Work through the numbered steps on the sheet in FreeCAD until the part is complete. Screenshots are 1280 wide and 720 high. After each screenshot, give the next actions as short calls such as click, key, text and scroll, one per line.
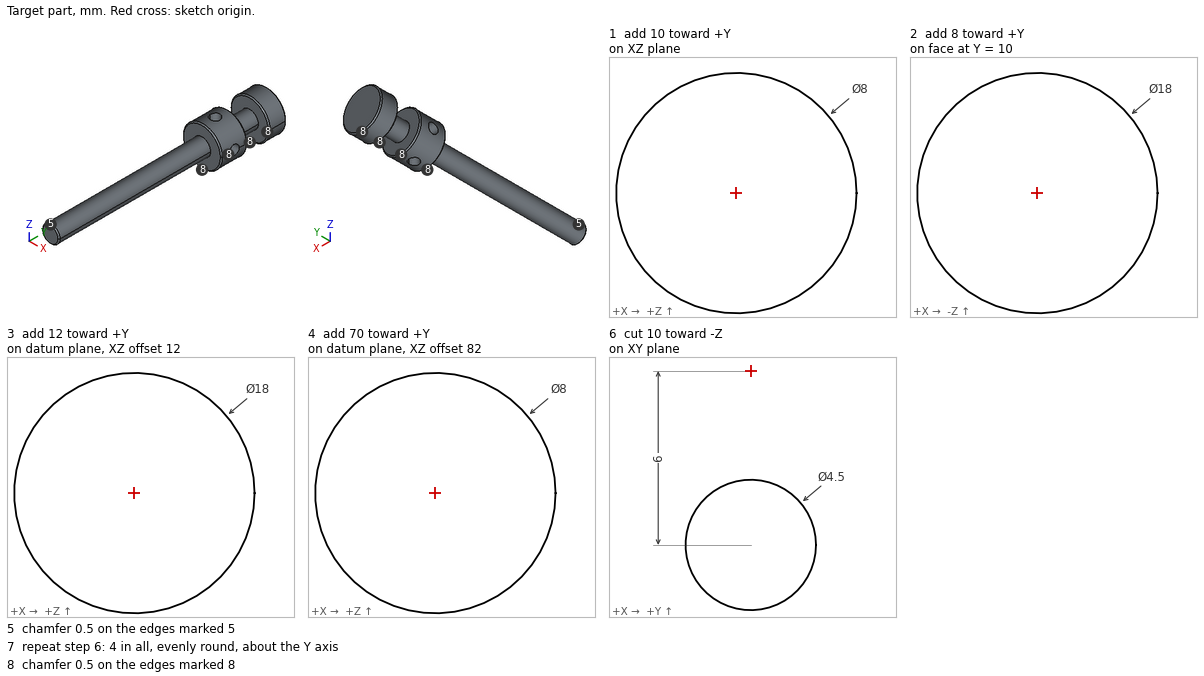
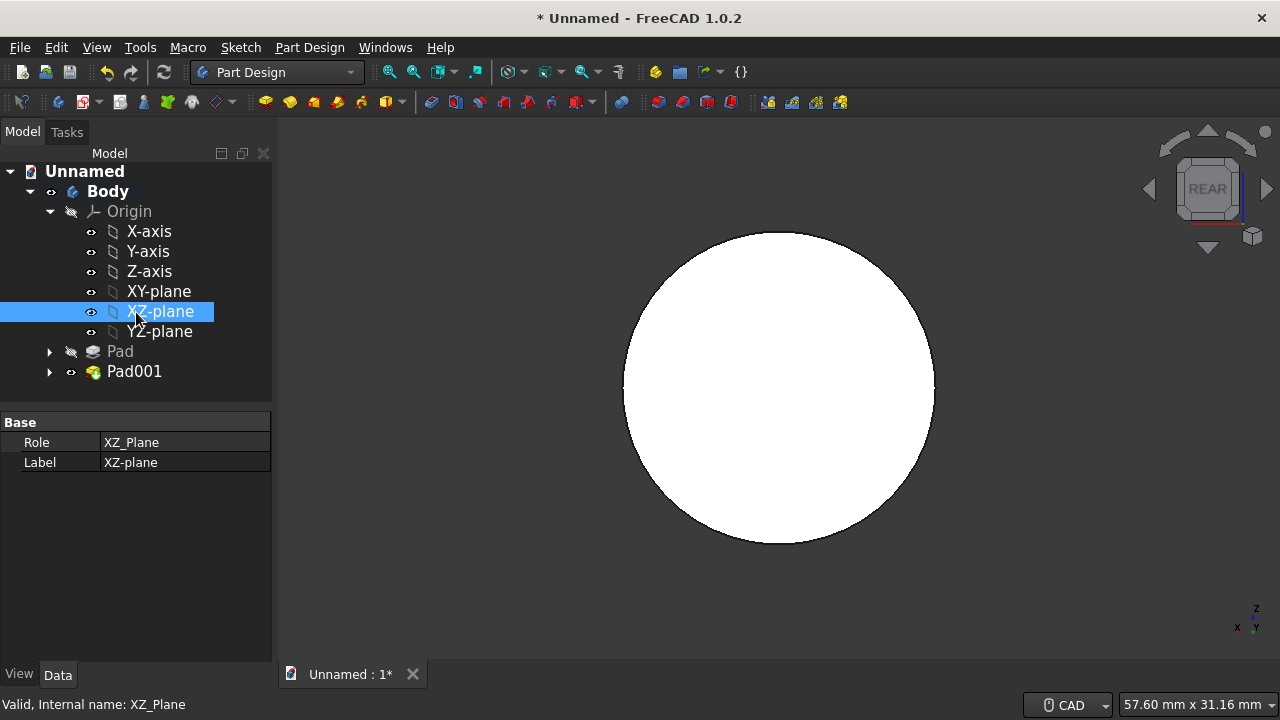
click(216, 102)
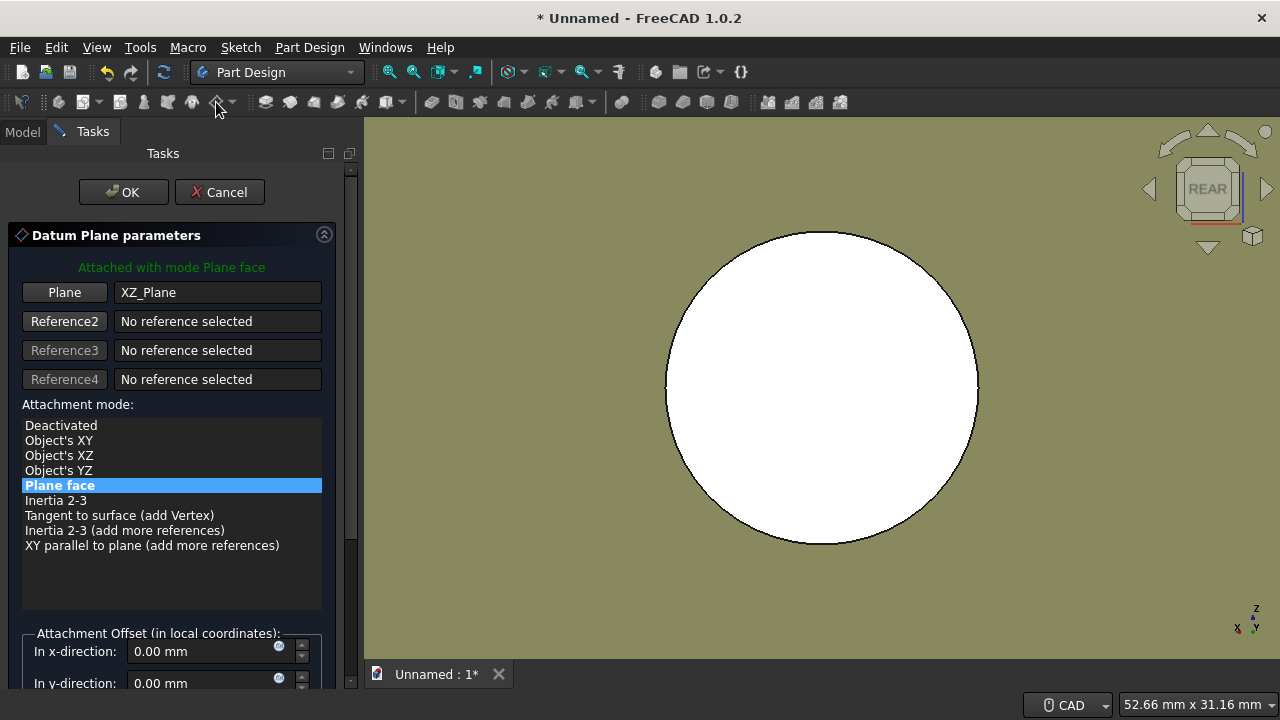
scroll(351, 426, down, 2)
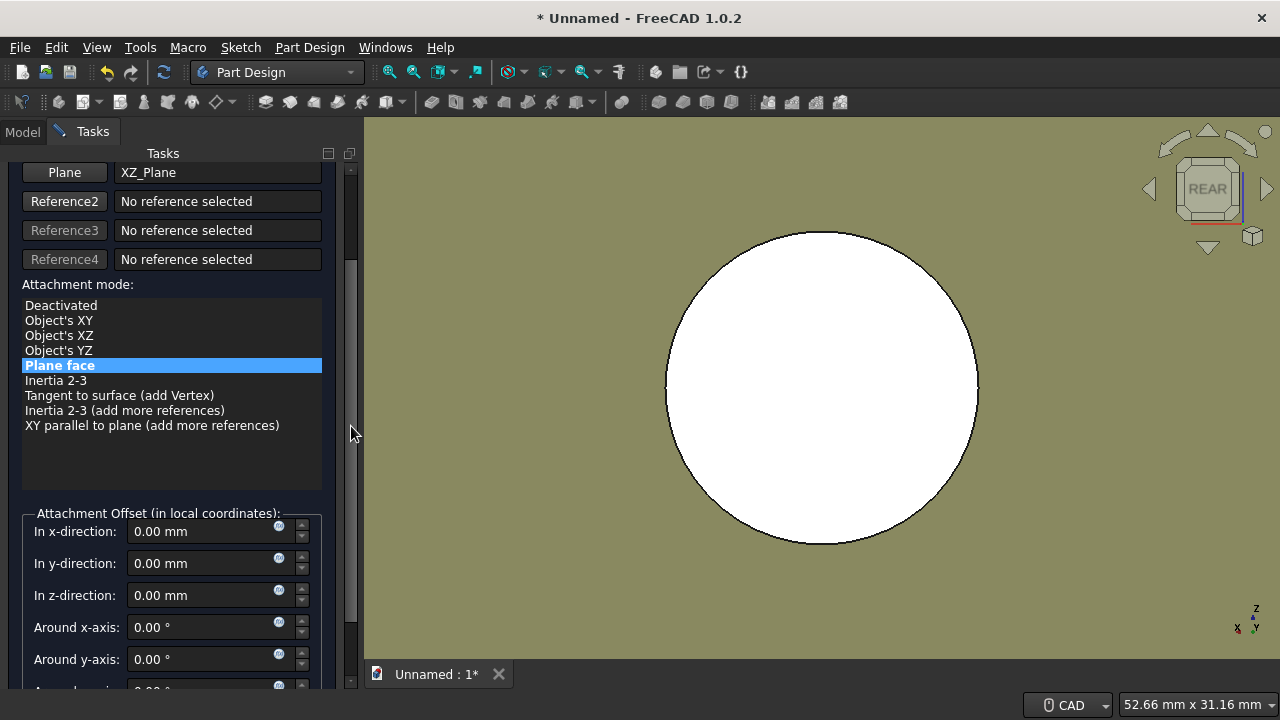
triple_click(210, 595)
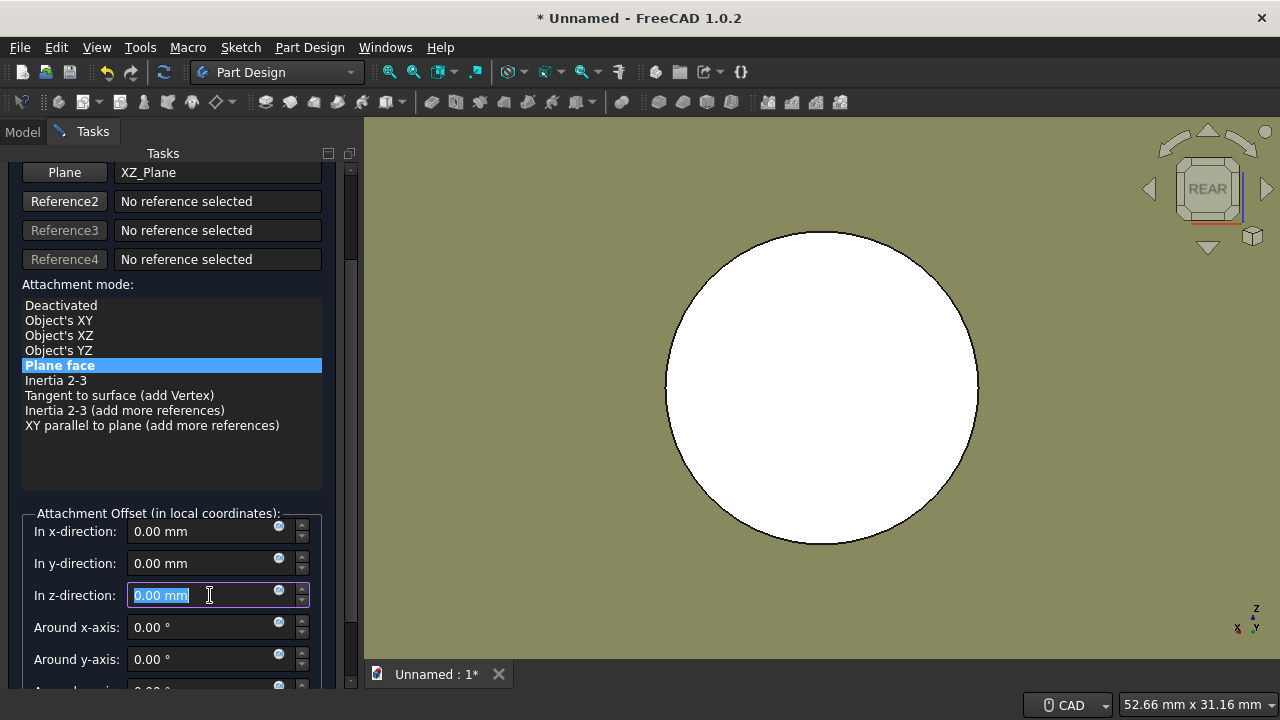
text(12)
key(Tab)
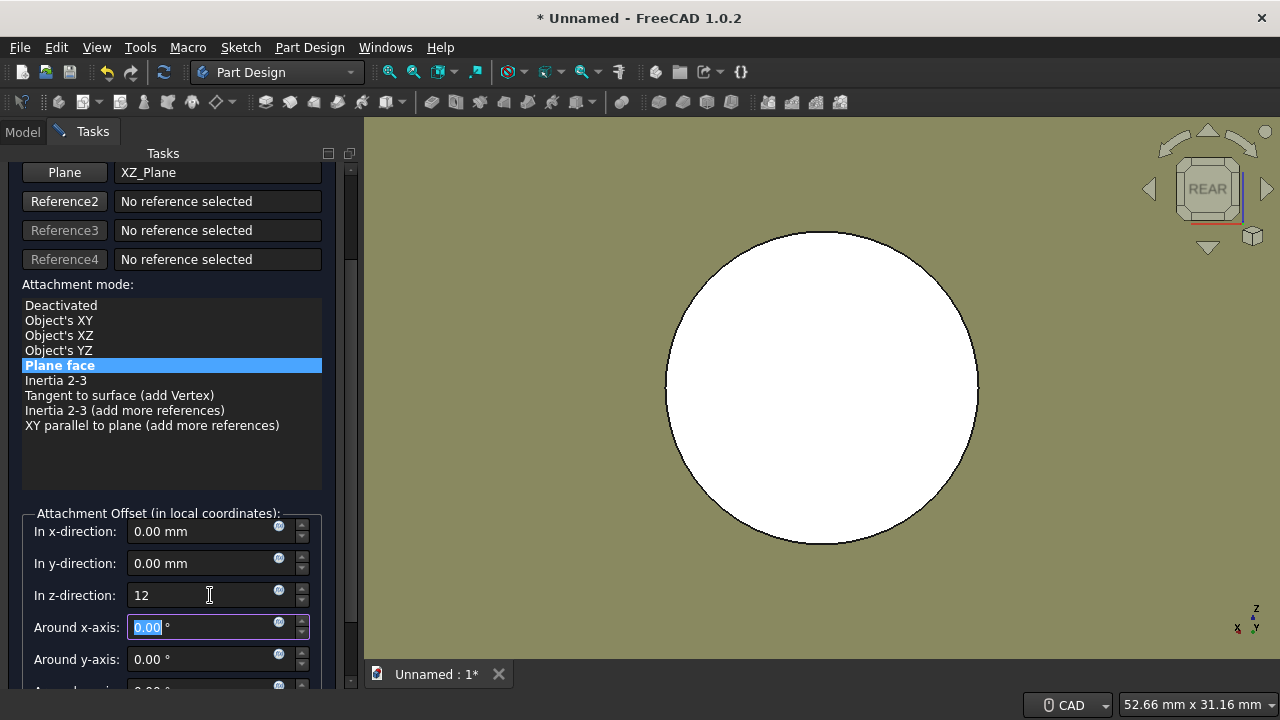
scroll(351, 426, up, 3)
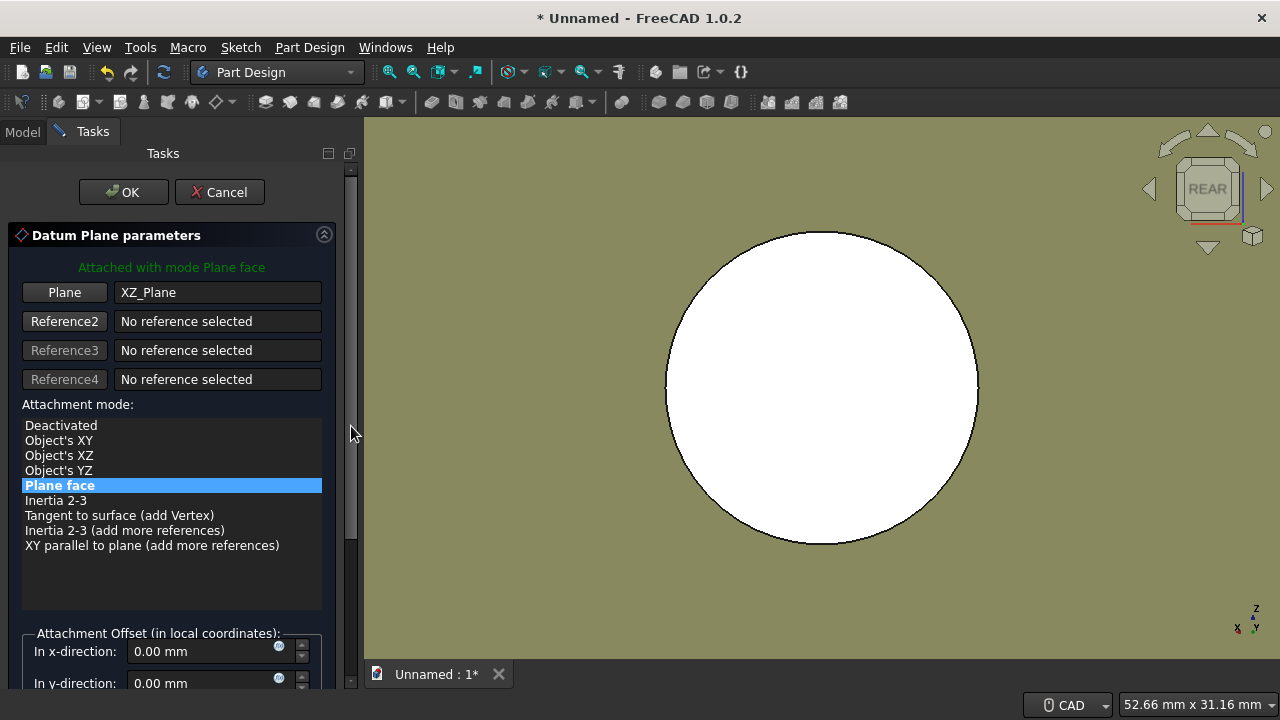
click(124, 192)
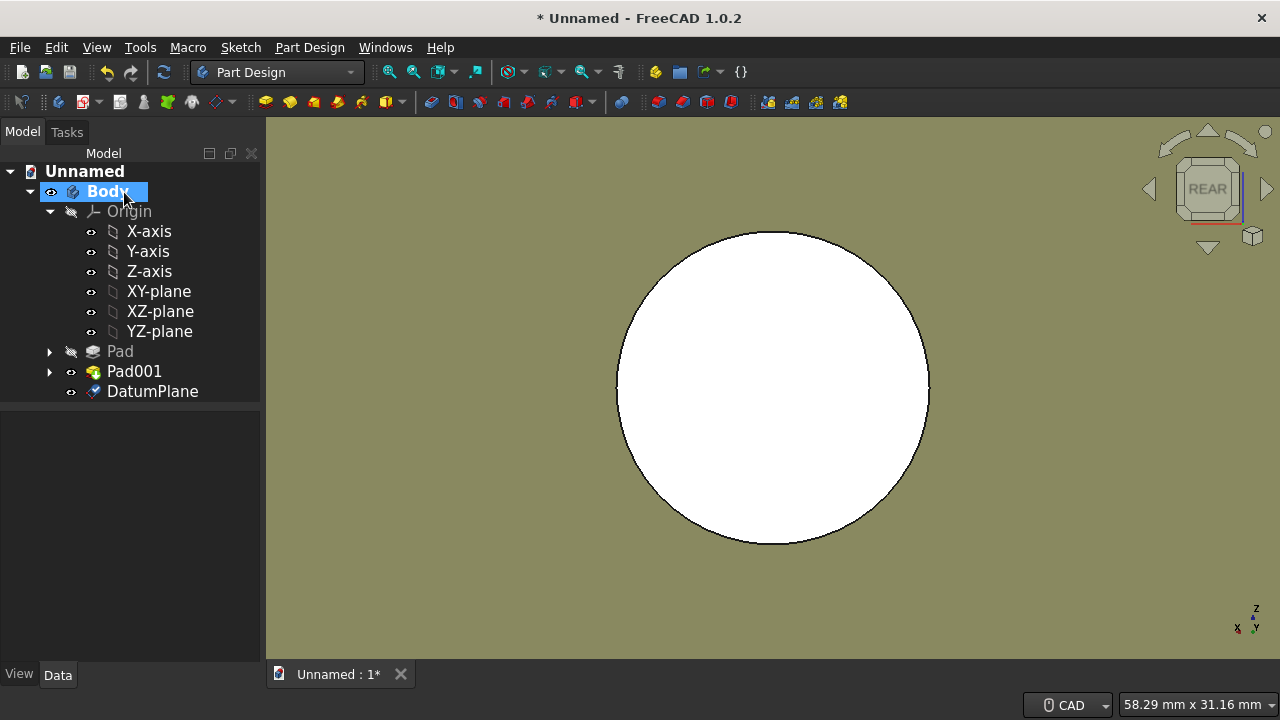
click(116, 392)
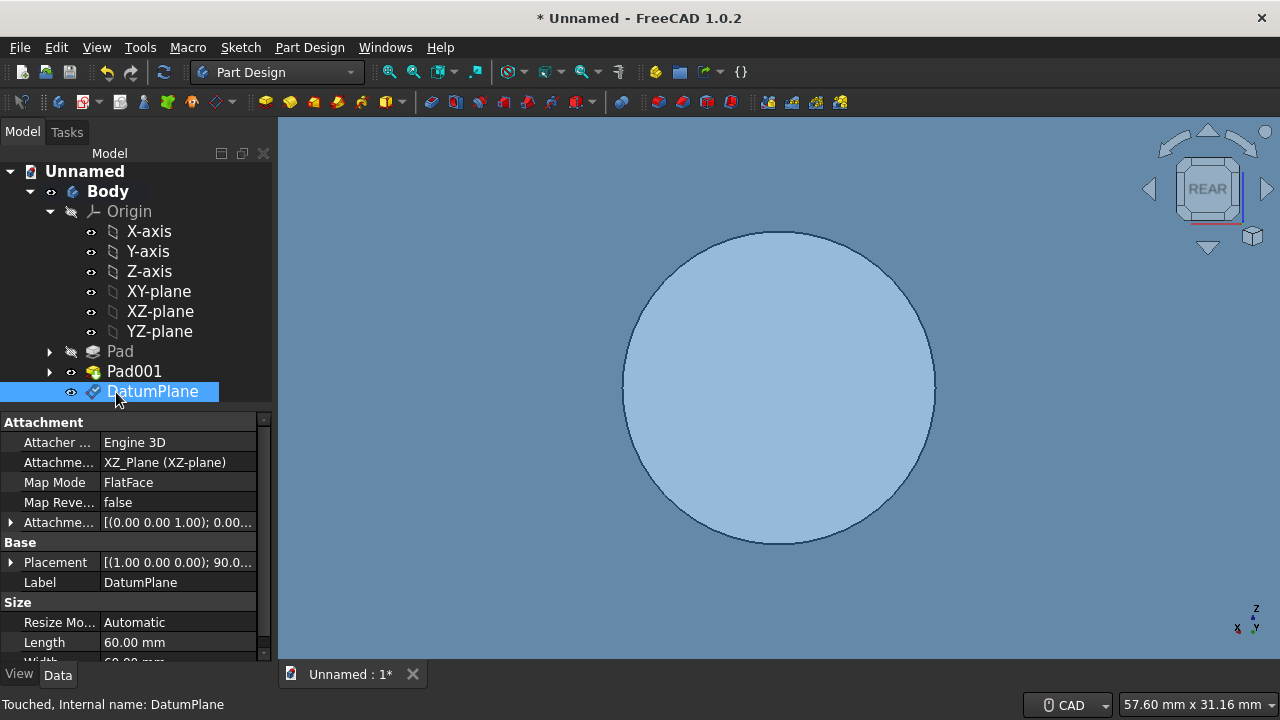
click(84, 102)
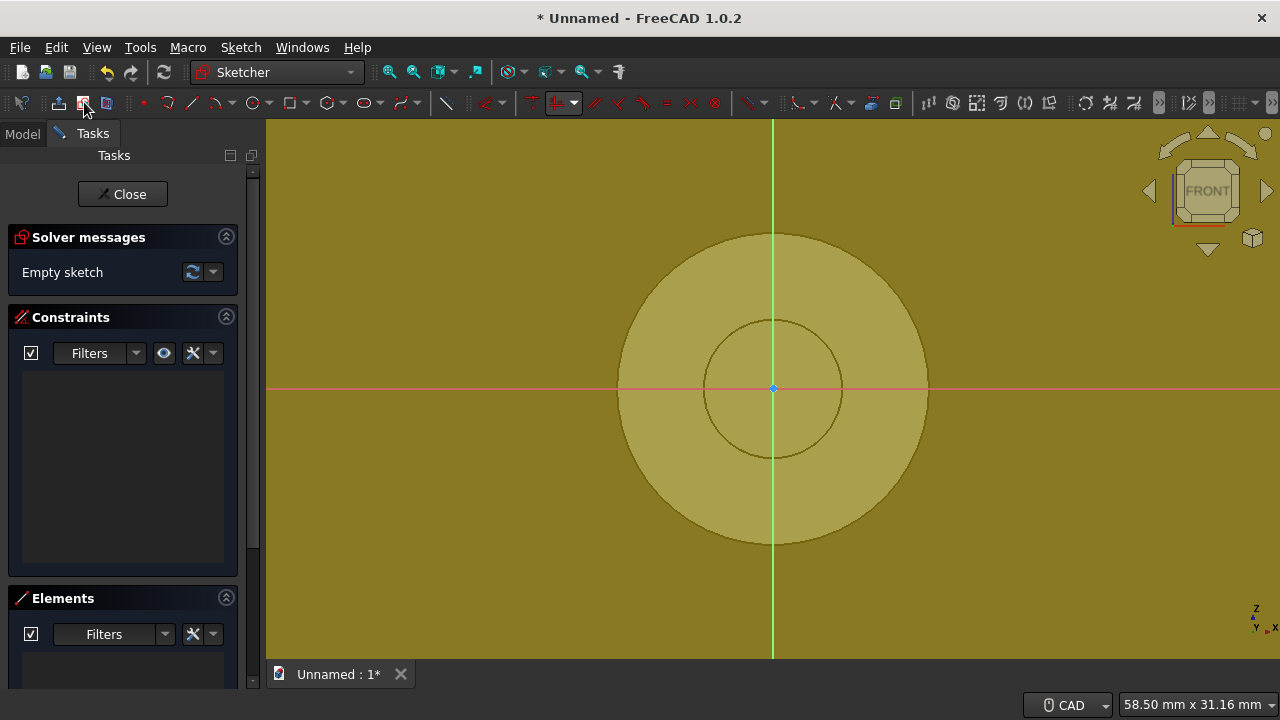
click(254, 104)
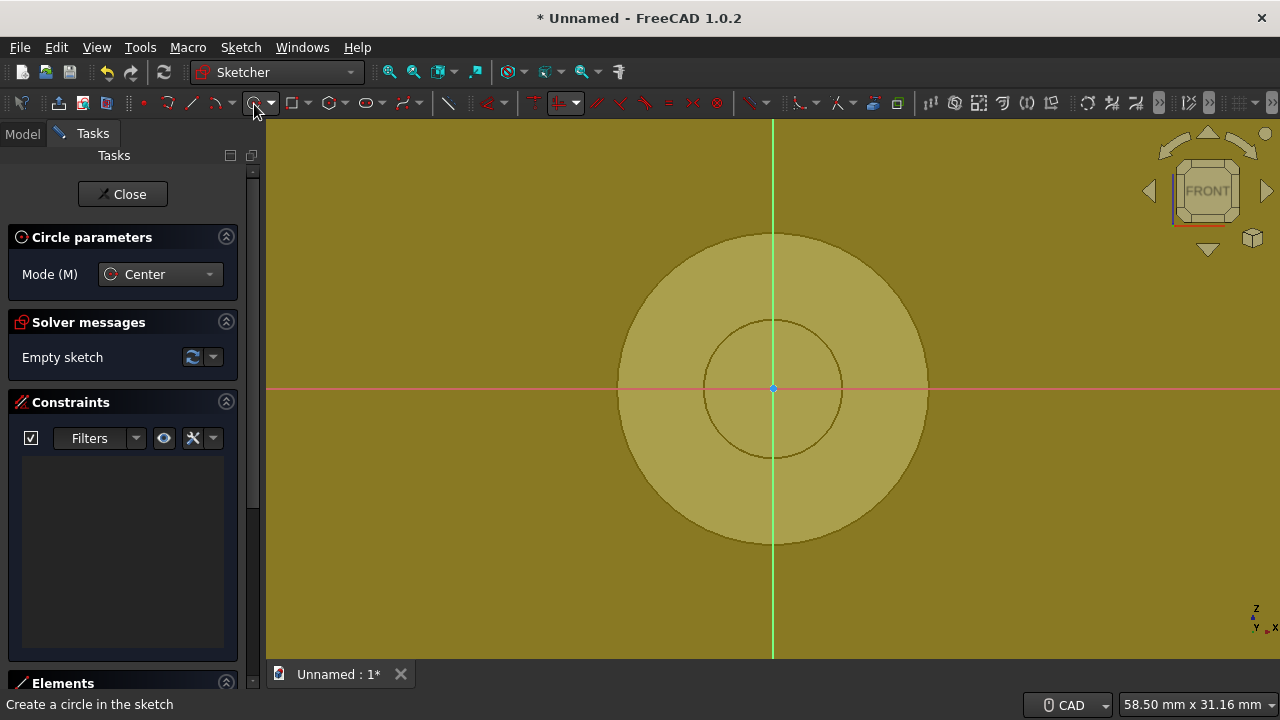
click(773, 389)
click(883, 279)
key(Escape)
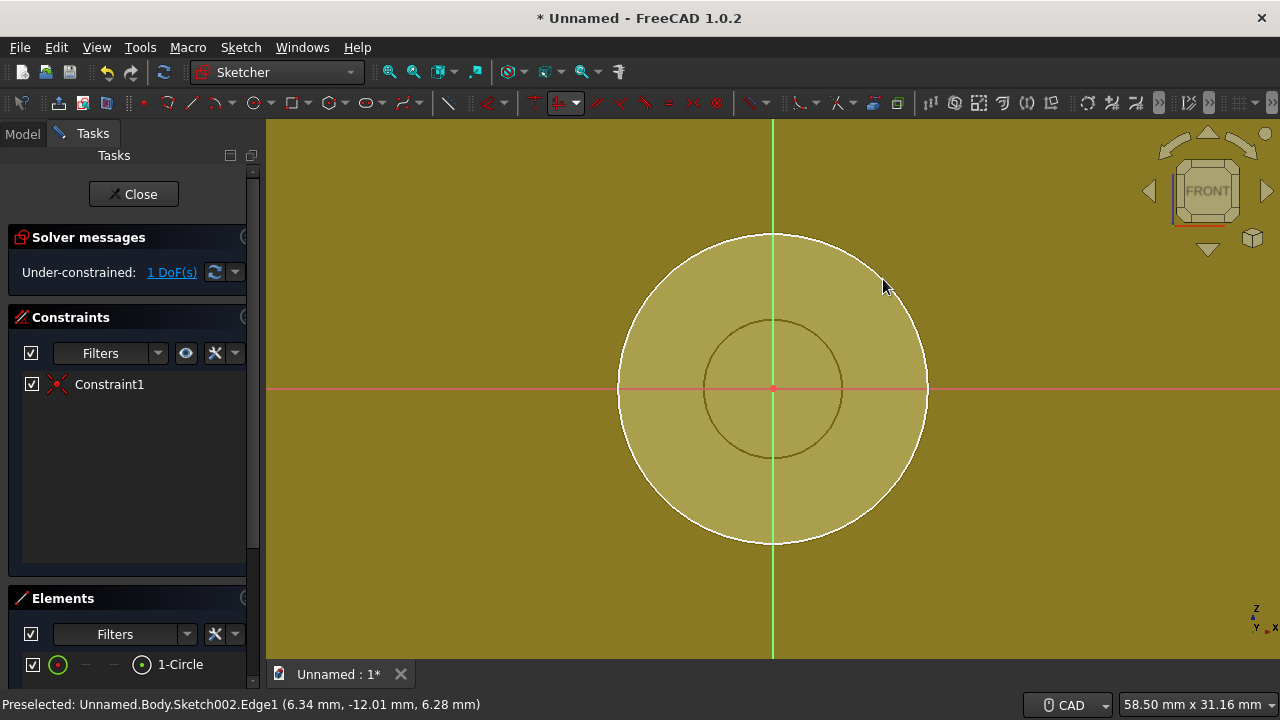
click(488, 104)